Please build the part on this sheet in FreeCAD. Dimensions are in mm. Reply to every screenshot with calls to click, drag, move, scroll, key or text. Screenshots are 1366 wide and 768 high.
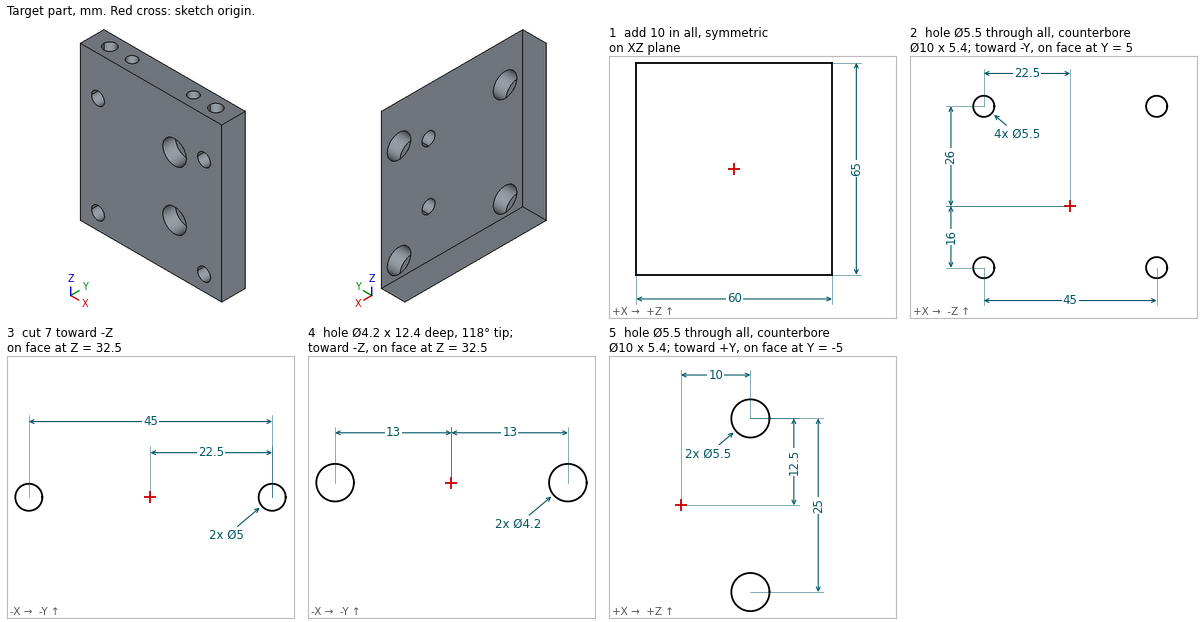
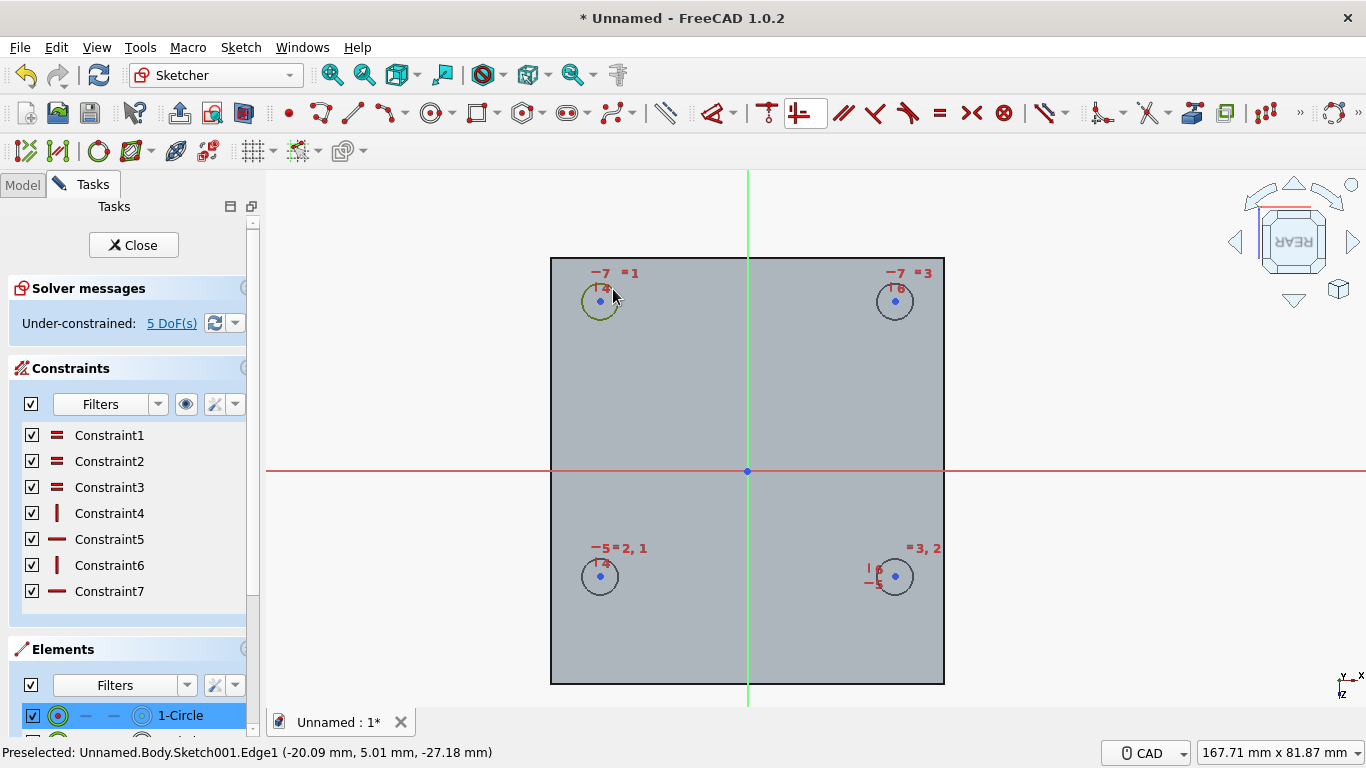
key(k)
key(o)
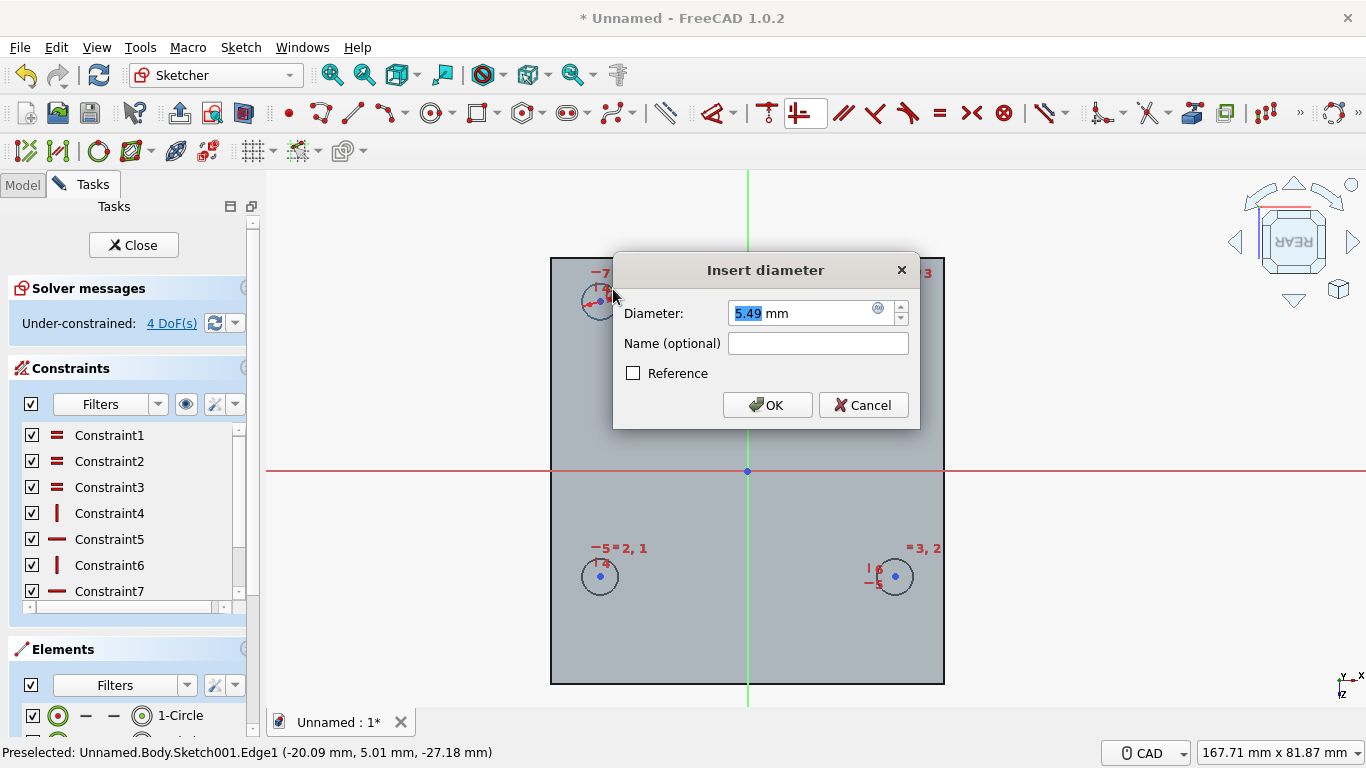
text(5.5)
key(Return)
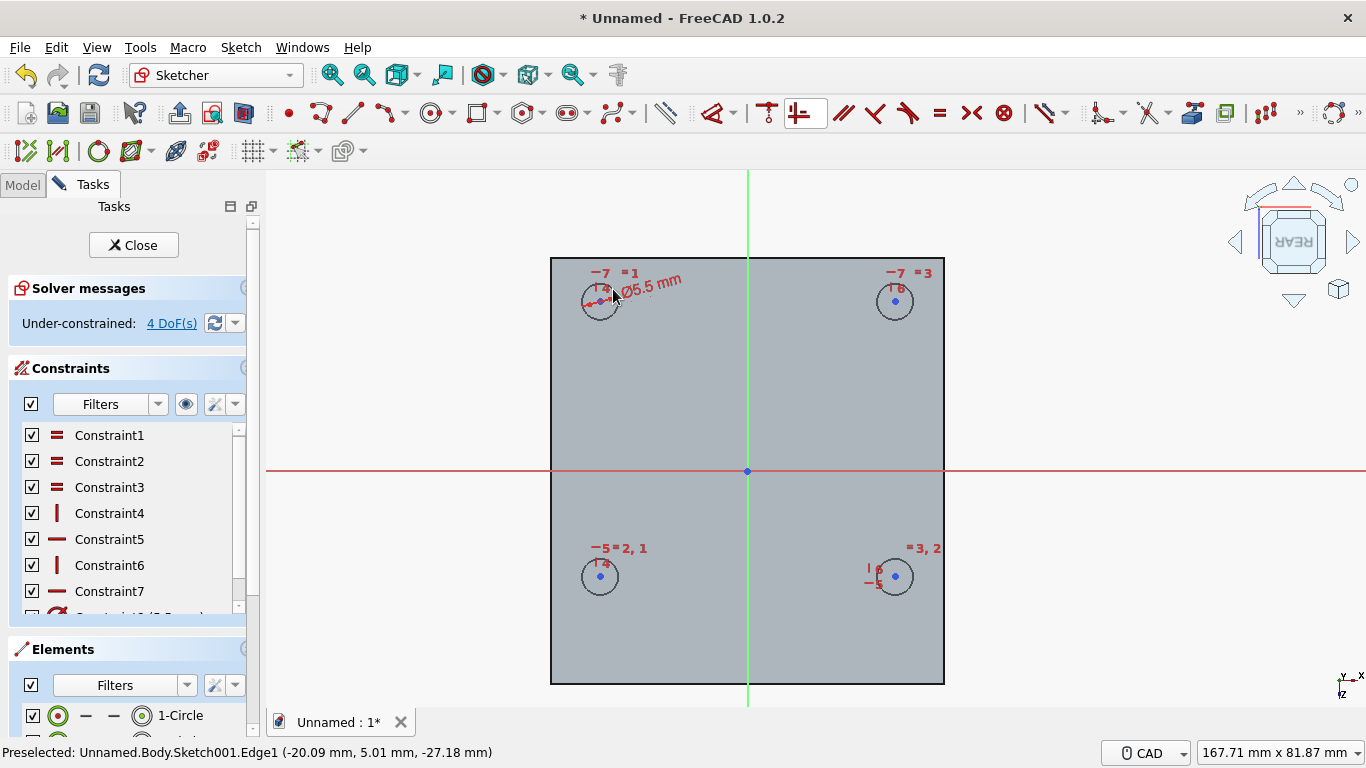
click(600, 302)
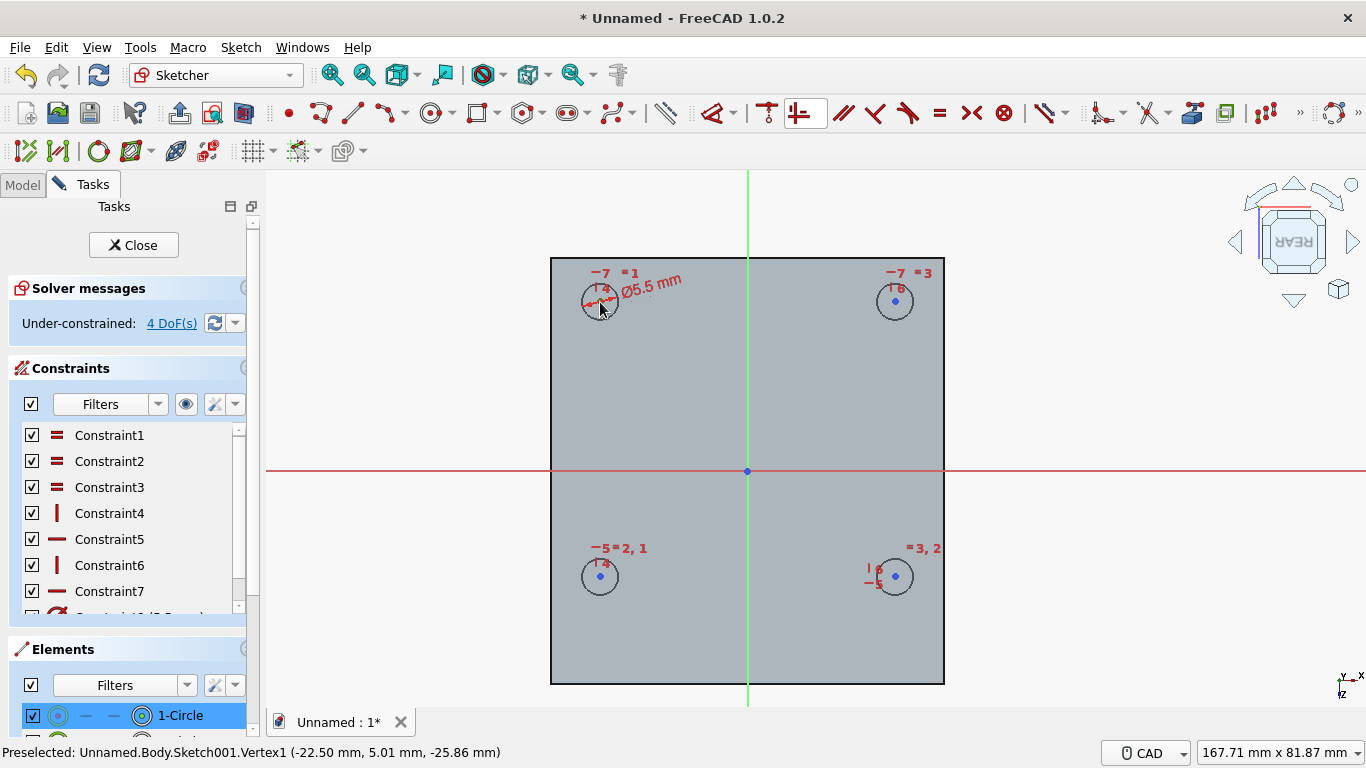
click(736, 114)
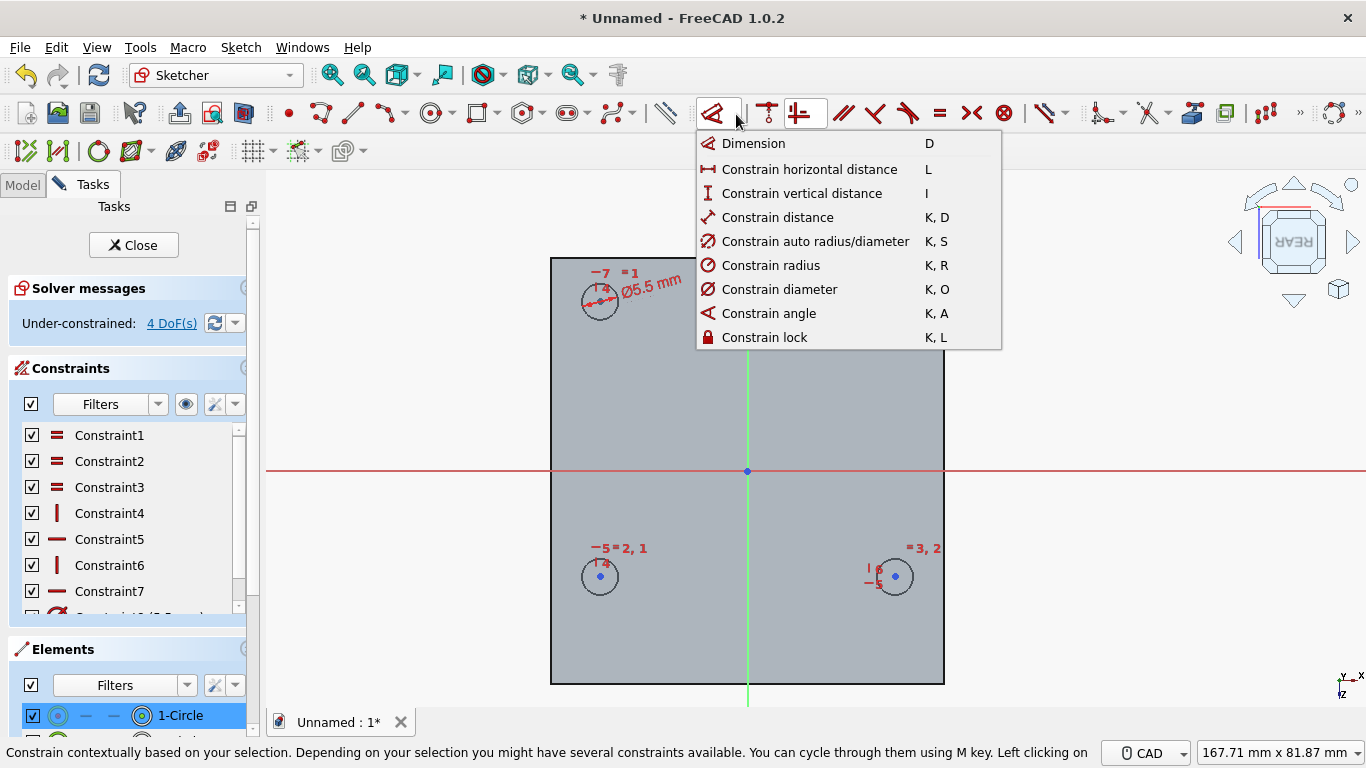
click(849, 193)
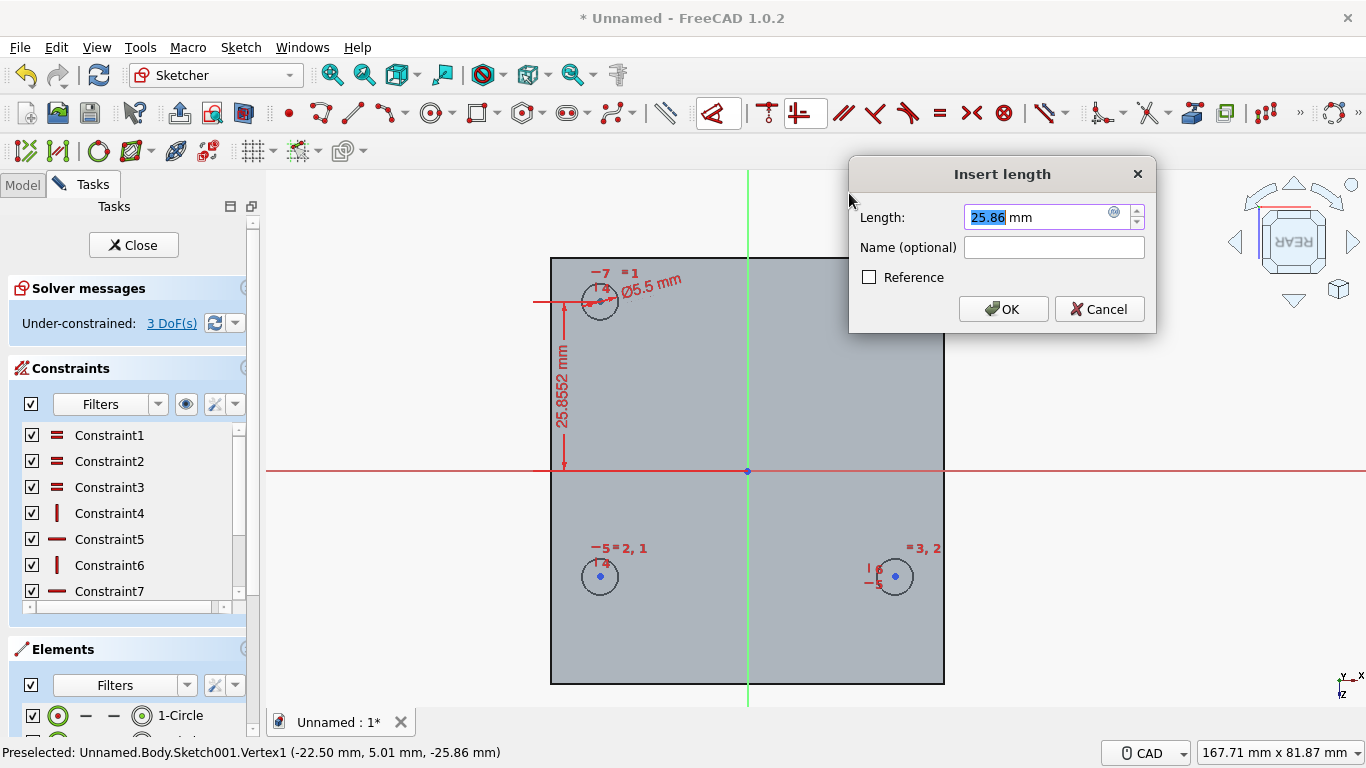
text(26)
key(Return)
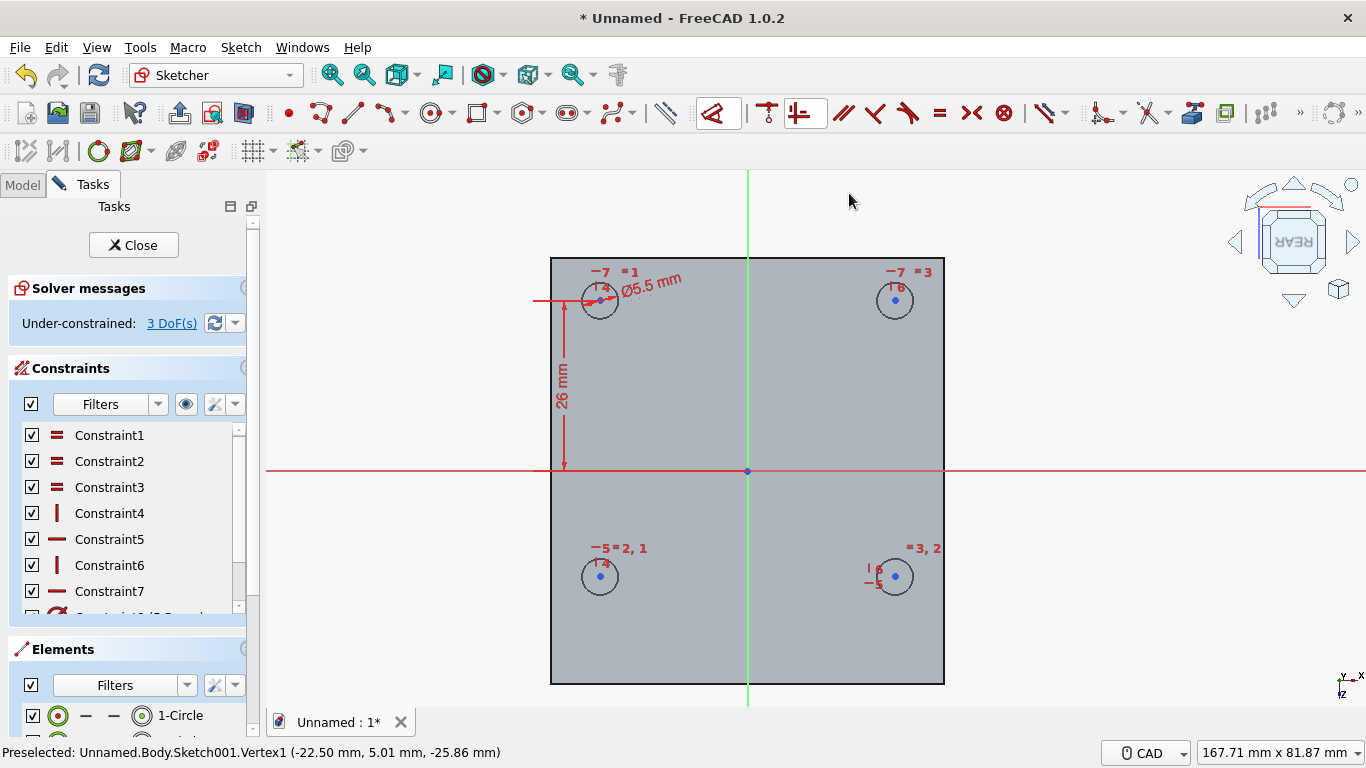
click(600, 577)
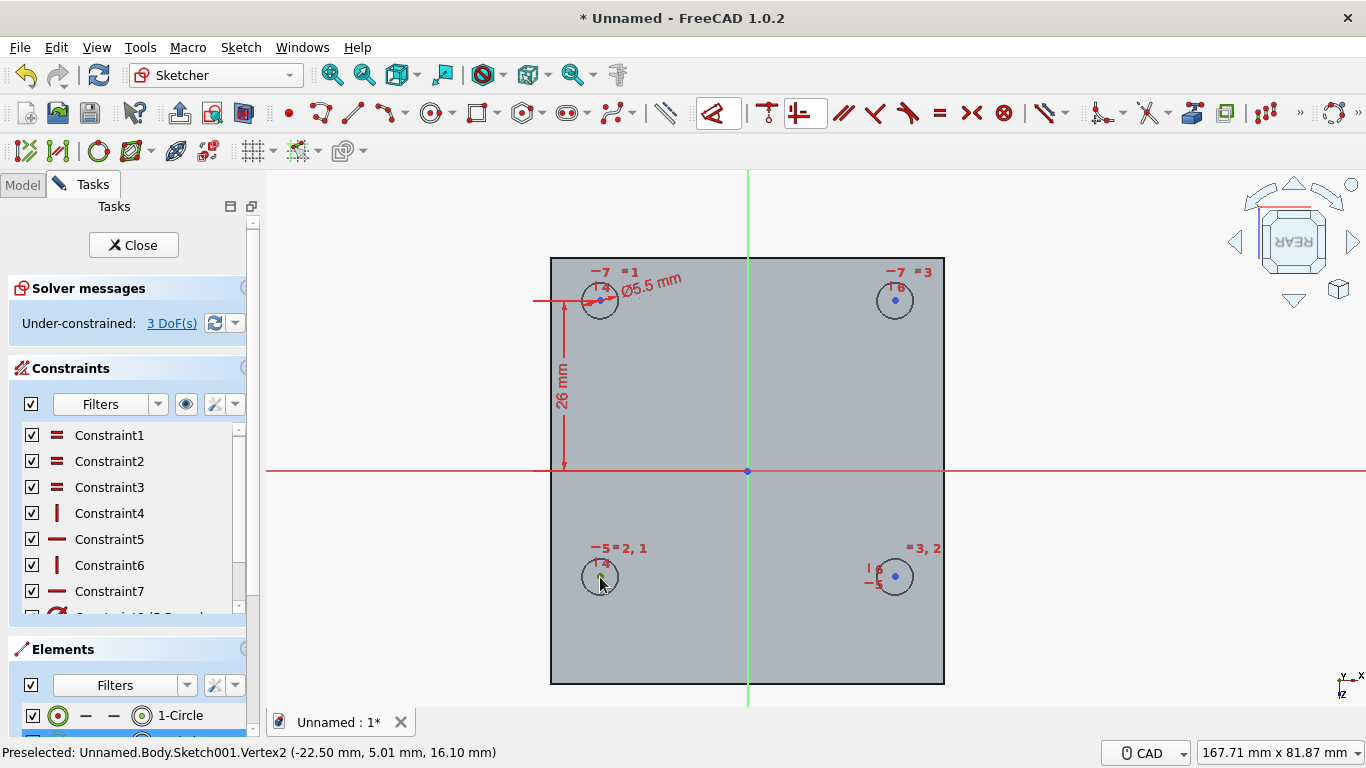
key(i)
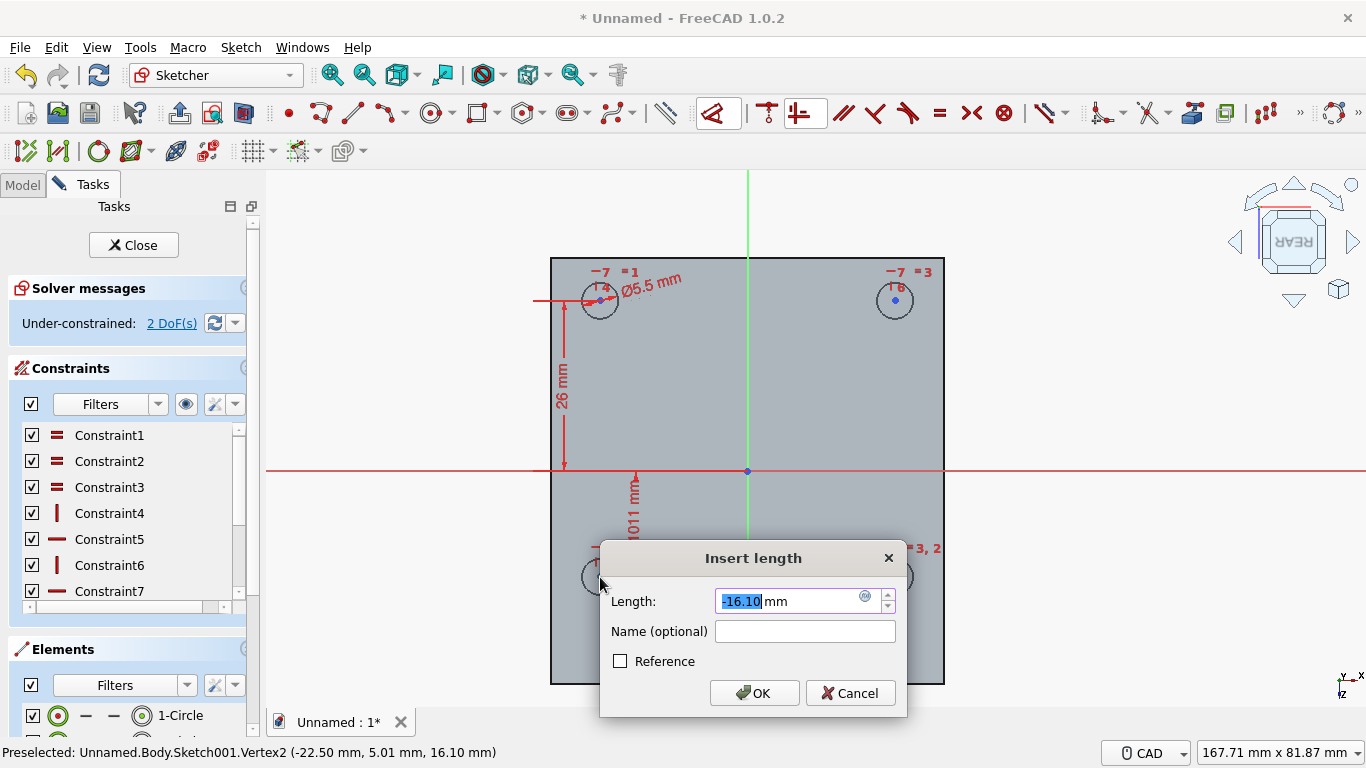
text(-16)
key(Return)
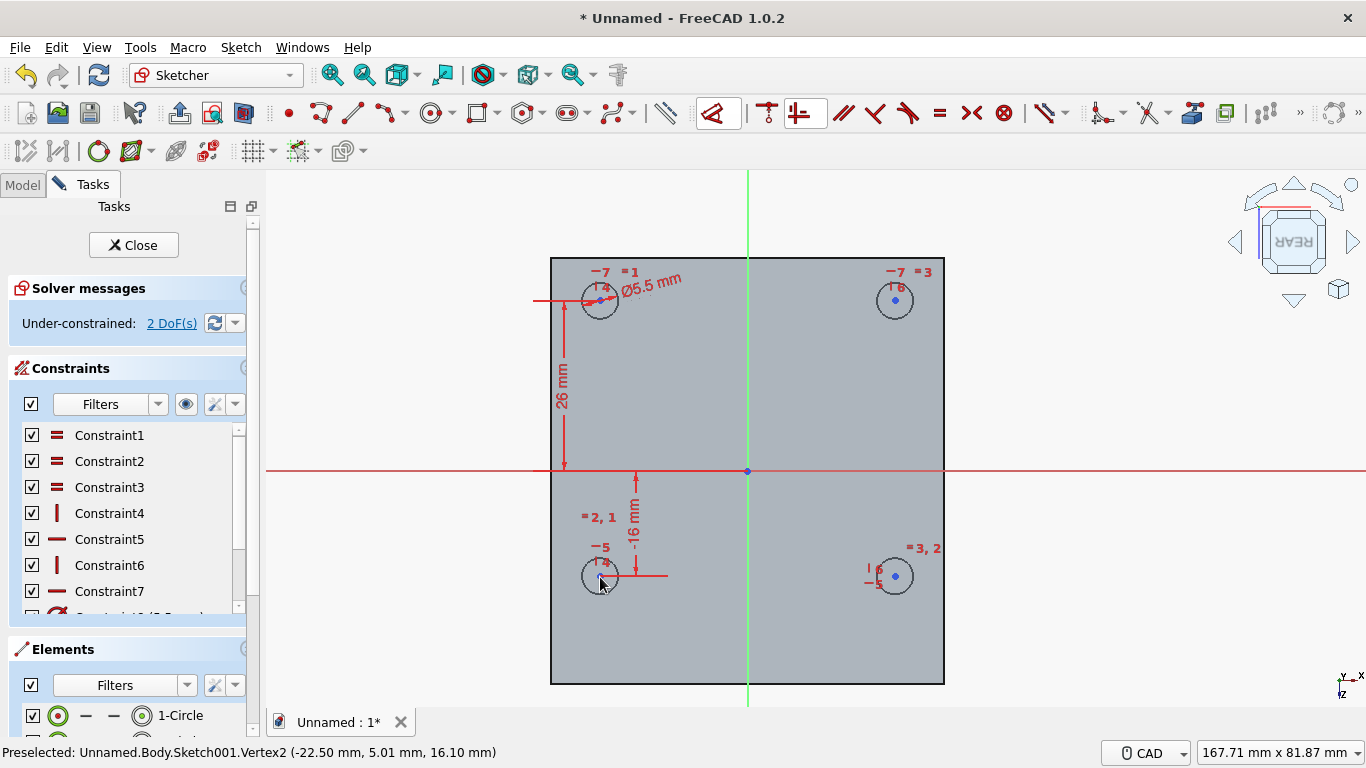
click(600, 576)